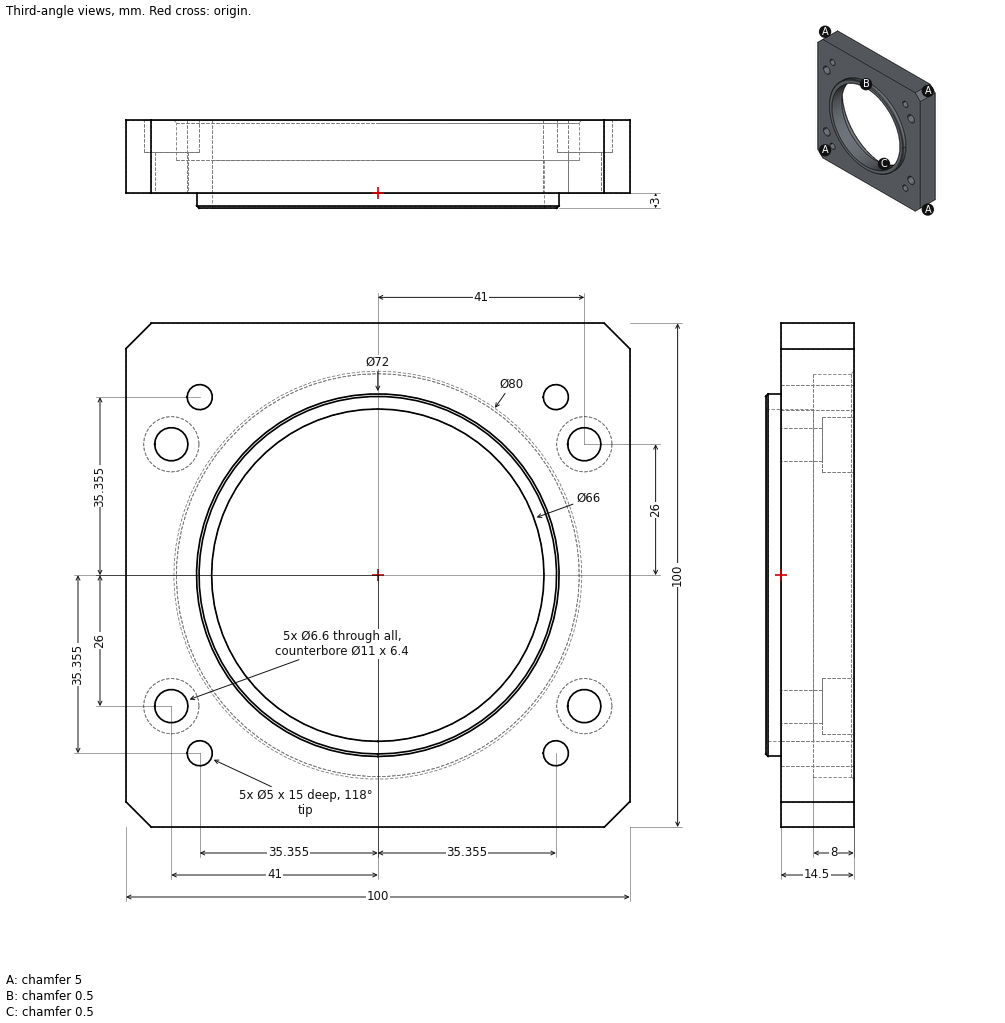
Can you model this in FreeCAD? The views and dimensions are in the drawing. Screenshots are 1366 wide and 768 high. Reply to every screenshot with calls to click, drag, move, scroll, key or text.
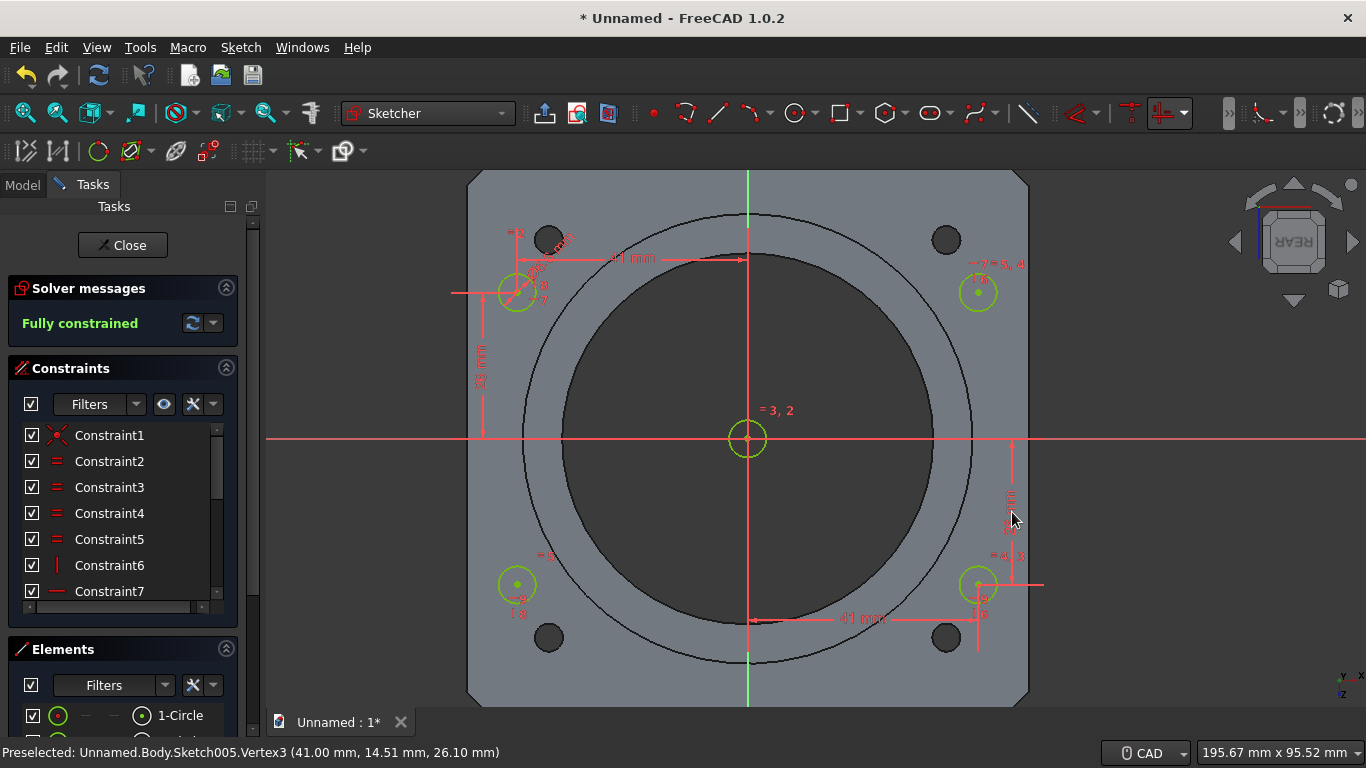
click(123, 245)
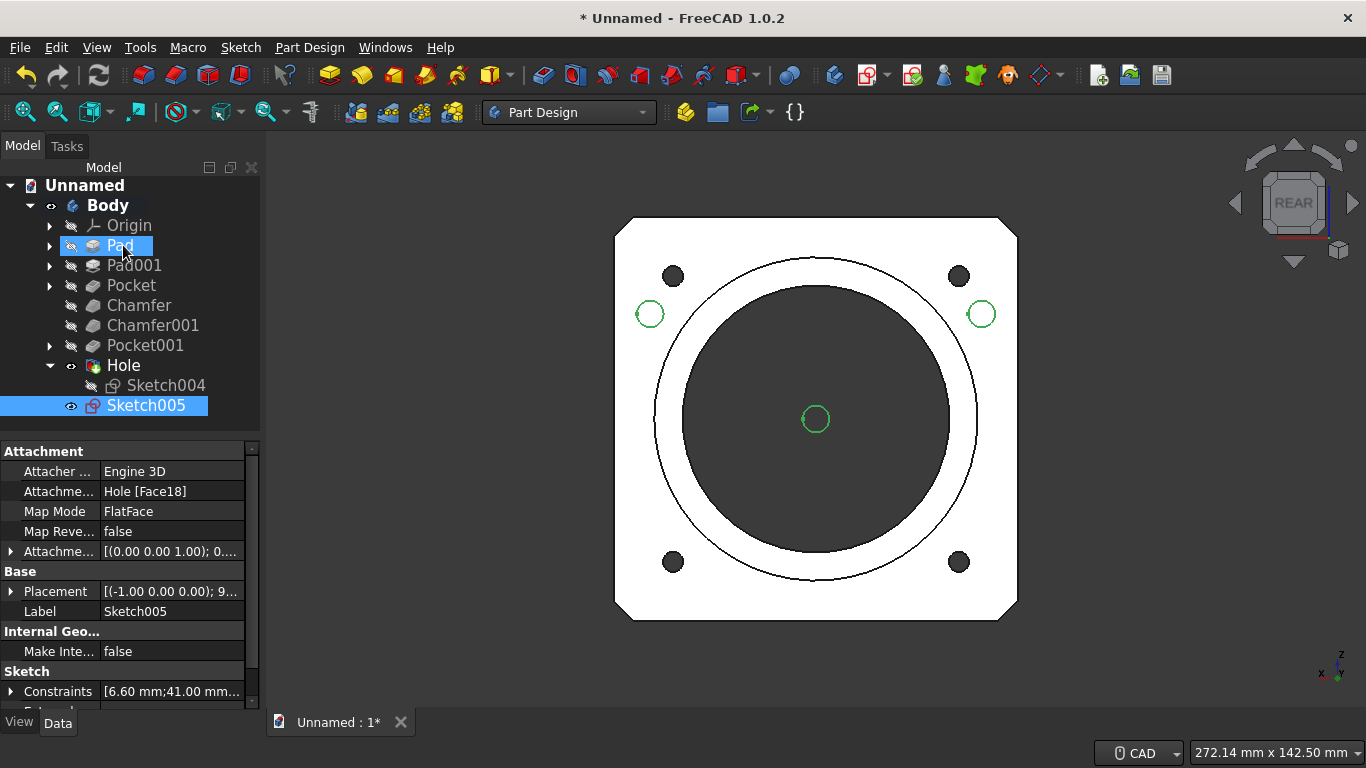
click(576, 76)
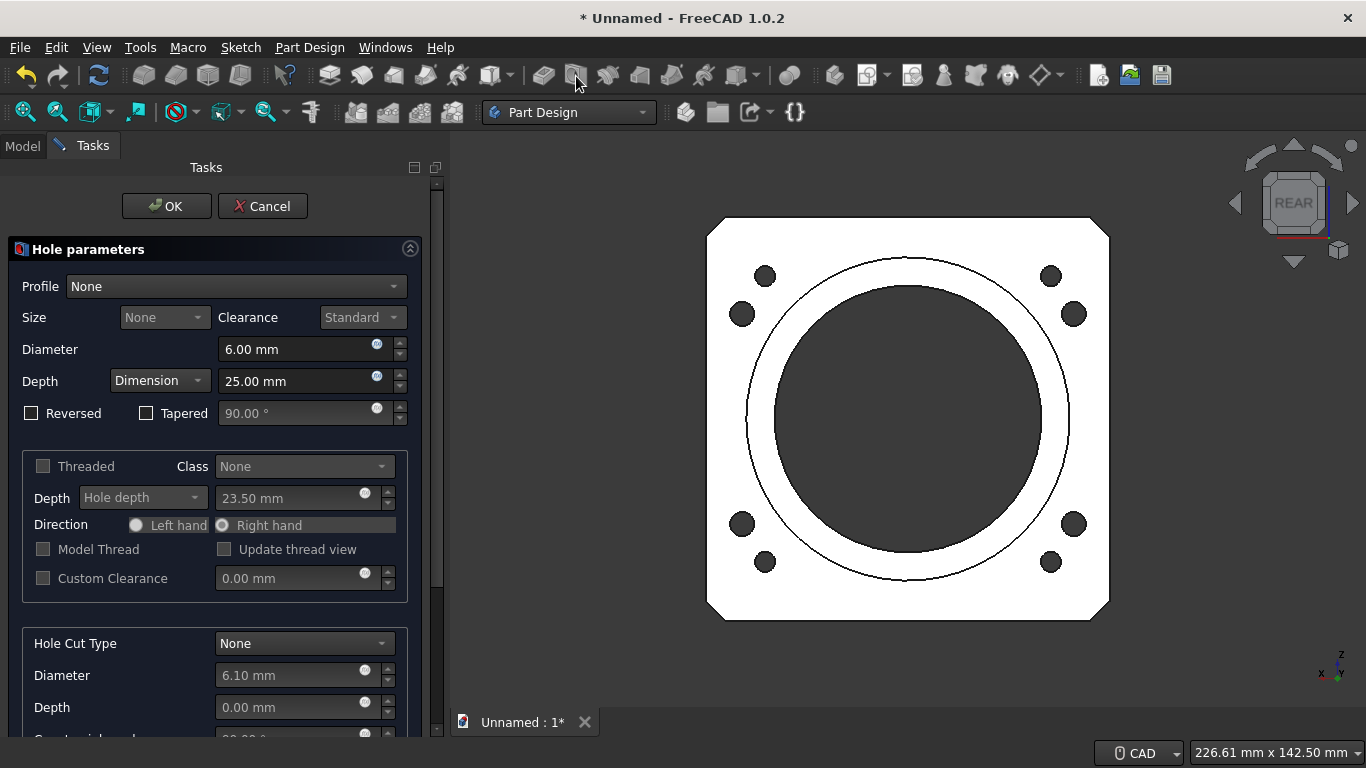
triple_click(305, 349)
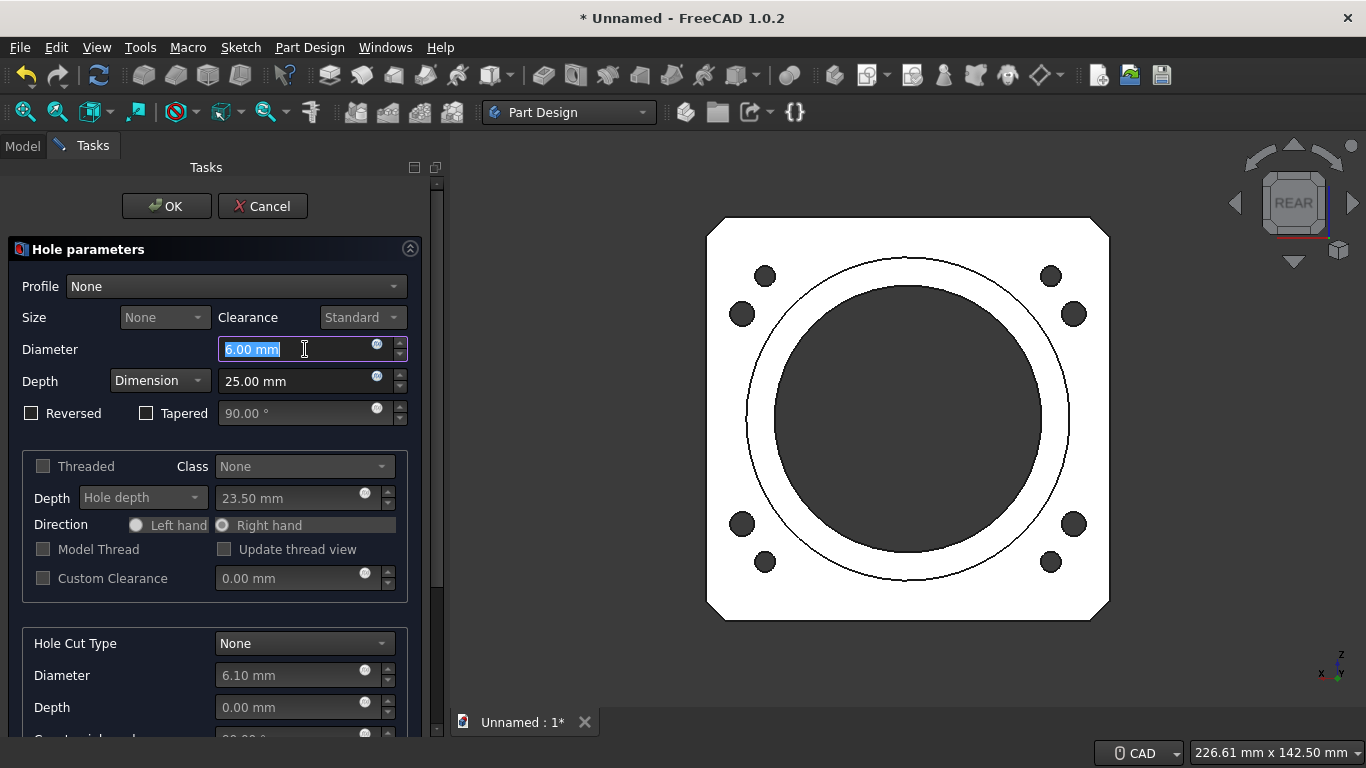
text(6.6)
key(Tab)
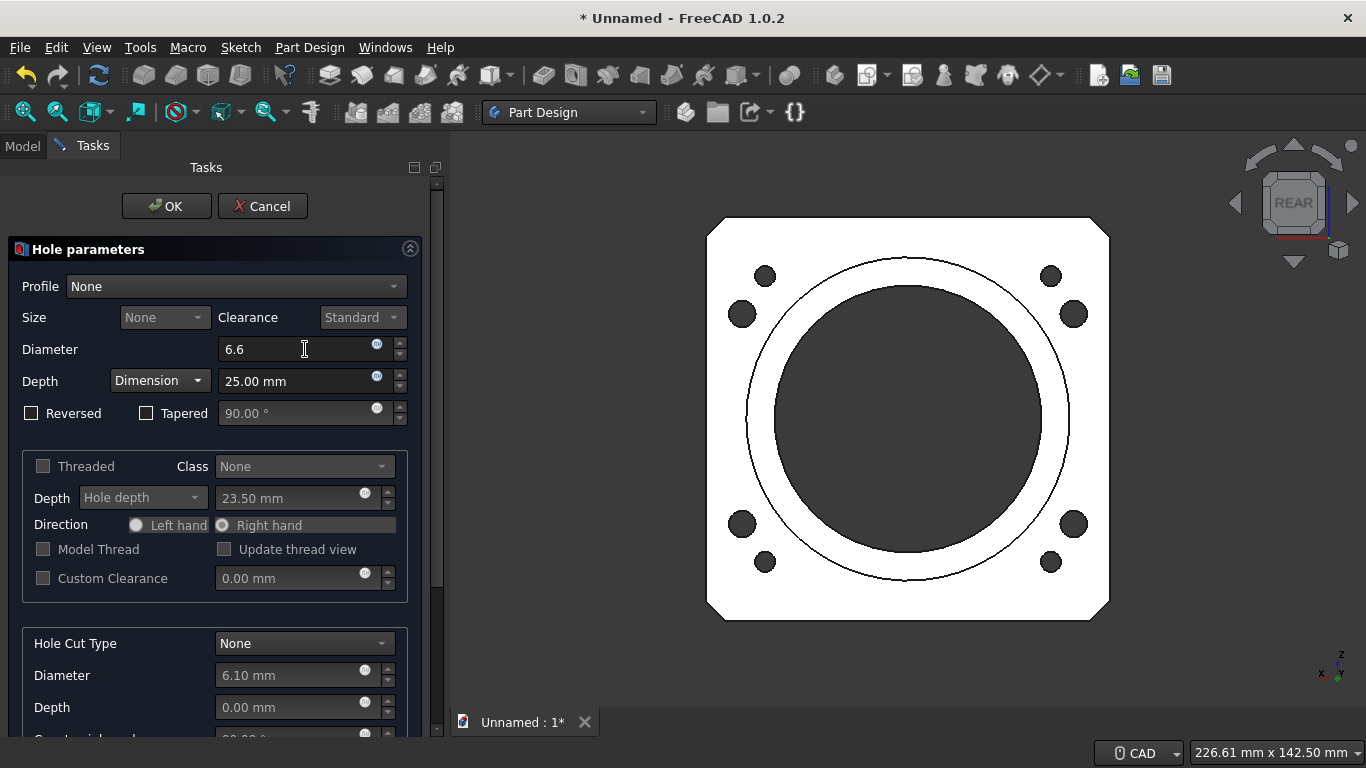
click(161, 380)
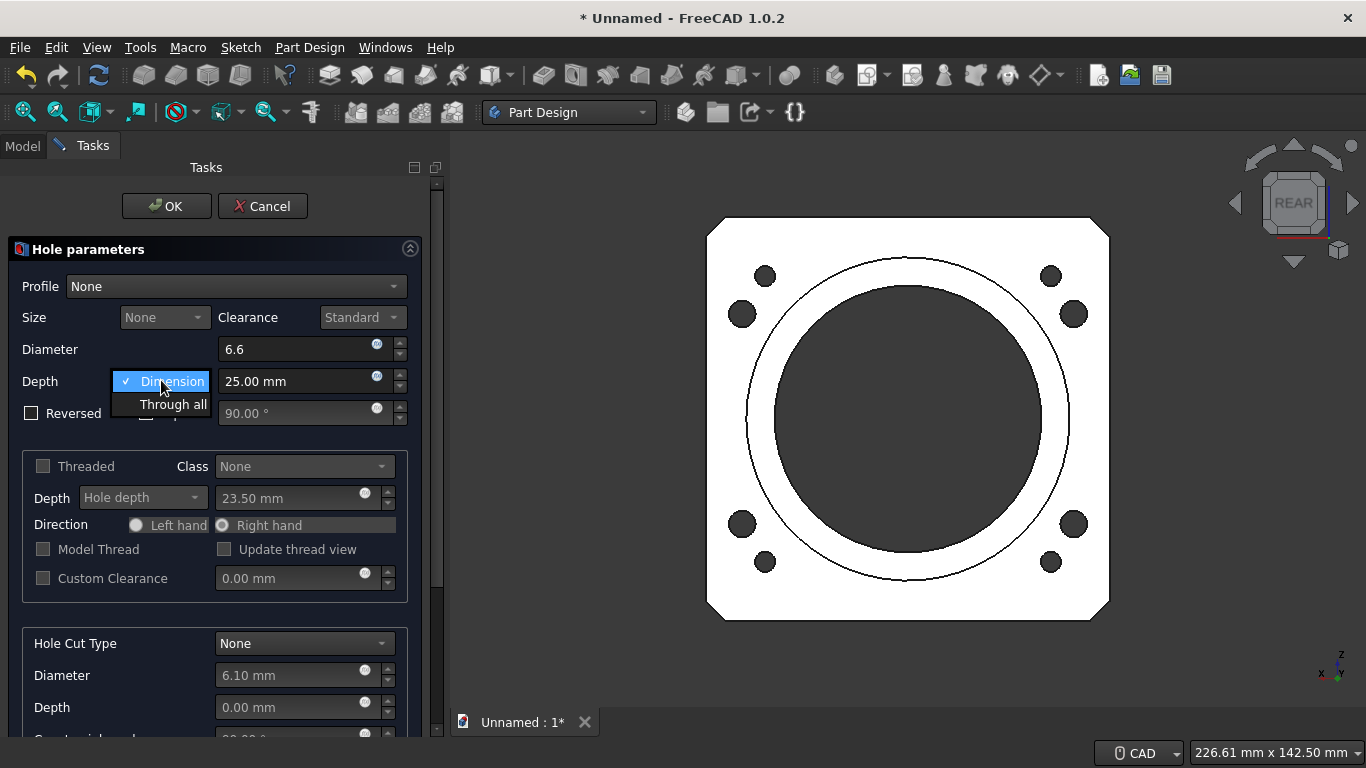
click(160, 404)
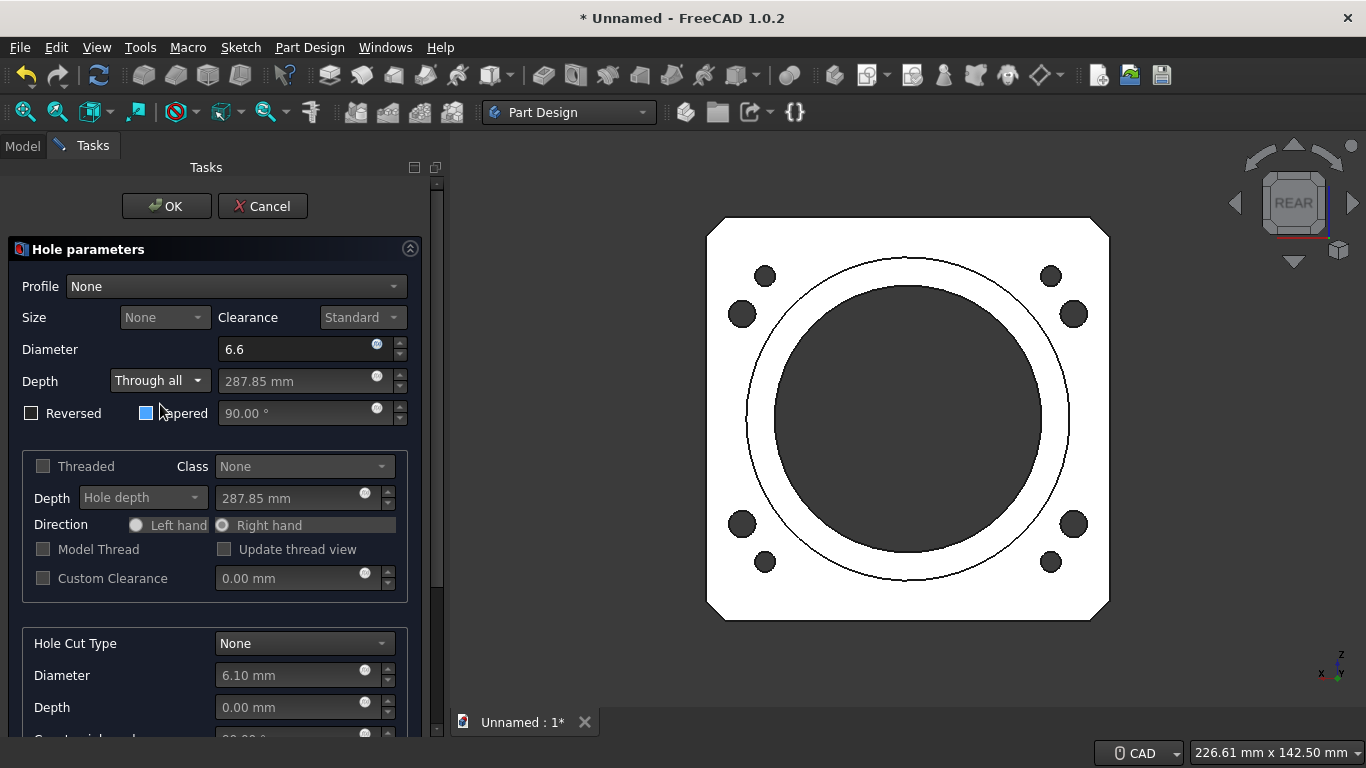
click(306, 644)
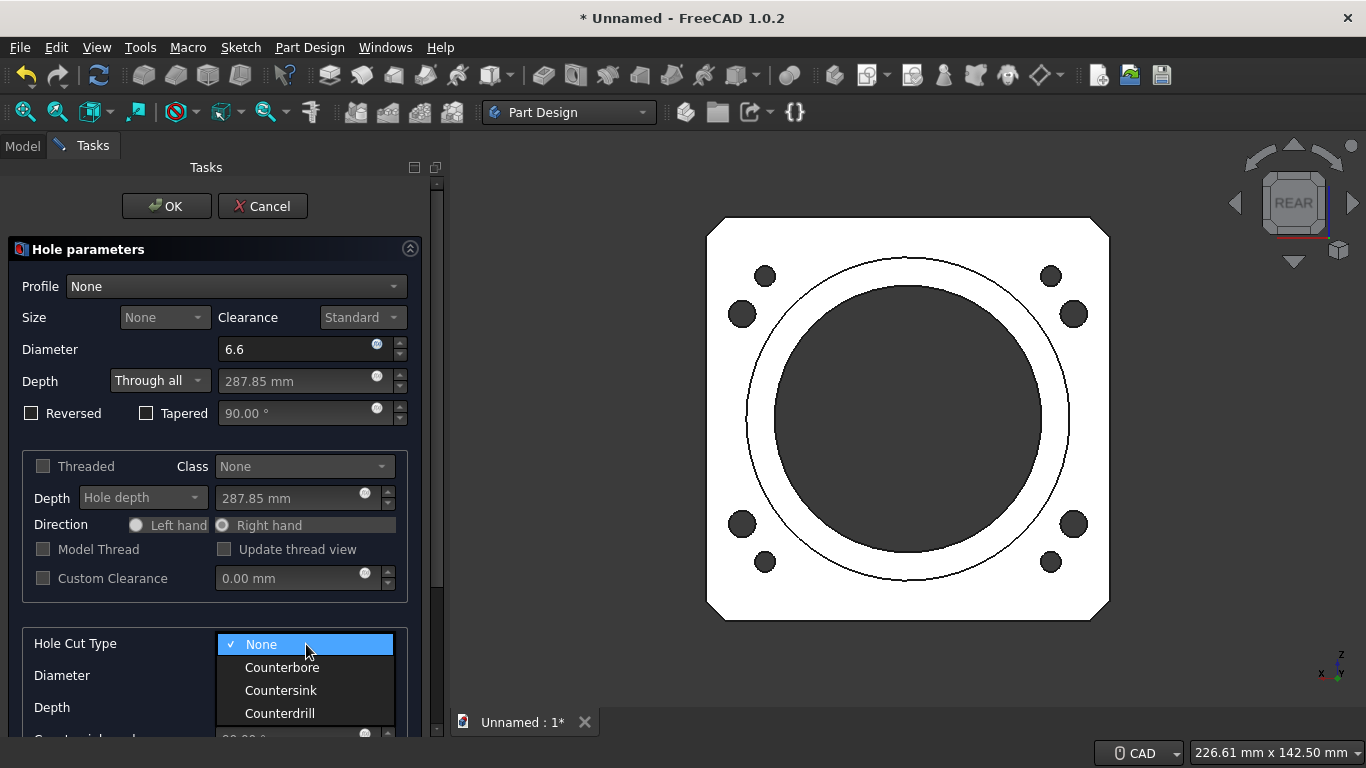
click(304, 668)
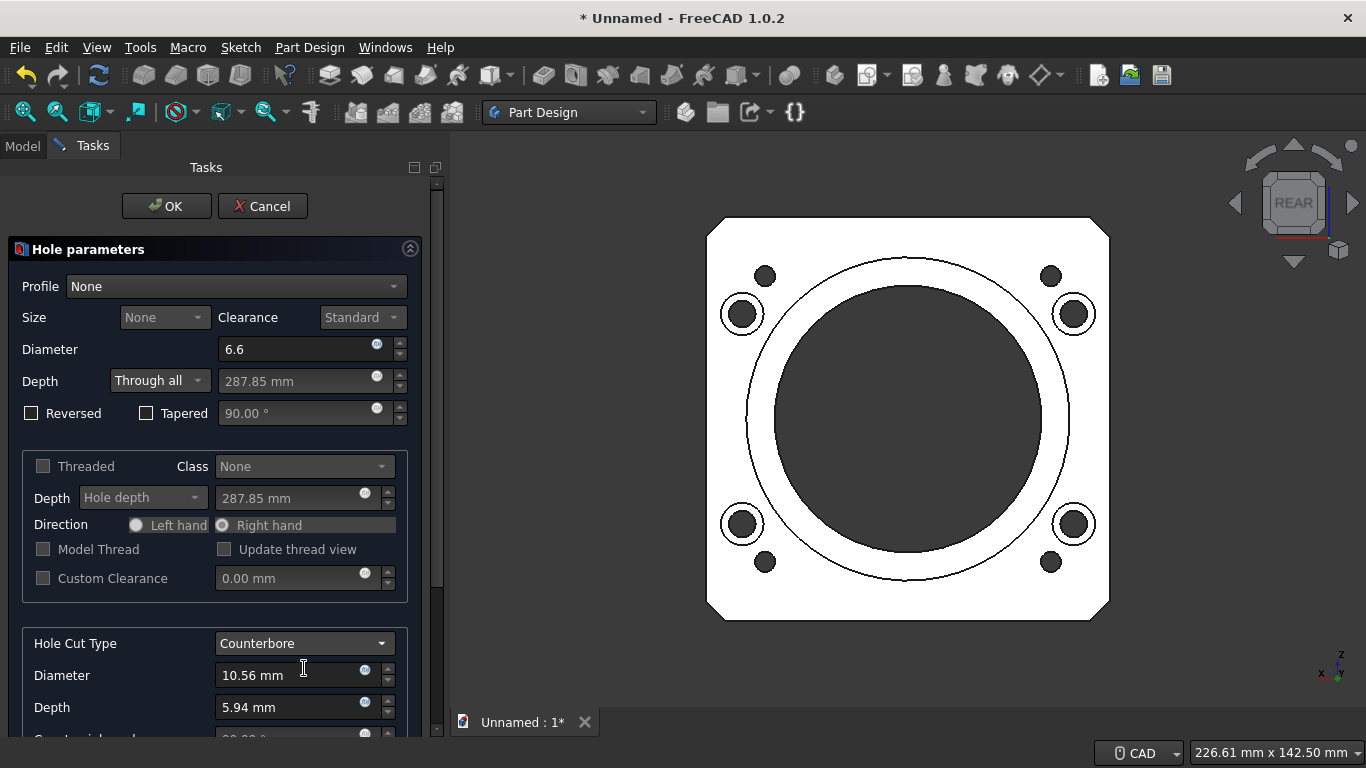
triple_click(298, 675)